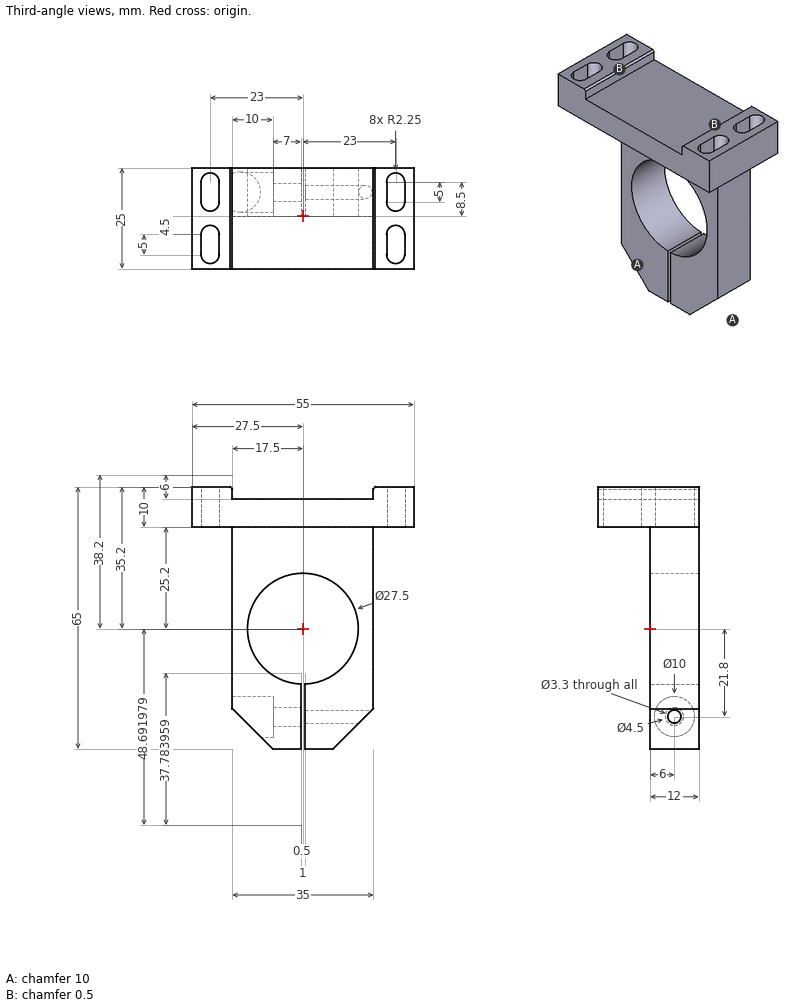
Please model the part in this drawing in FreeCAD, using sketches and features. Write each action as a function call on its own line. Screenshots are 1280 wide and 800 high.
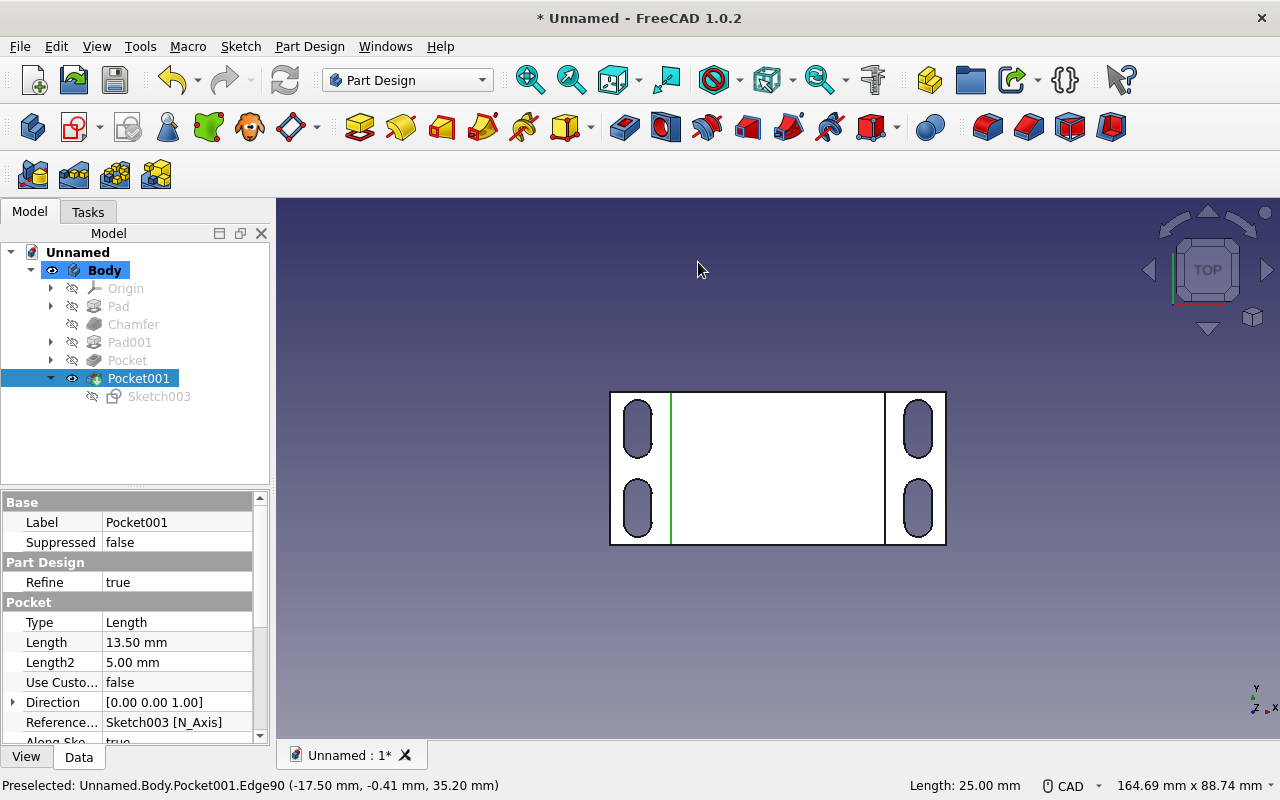
click(885, 467, ctrl)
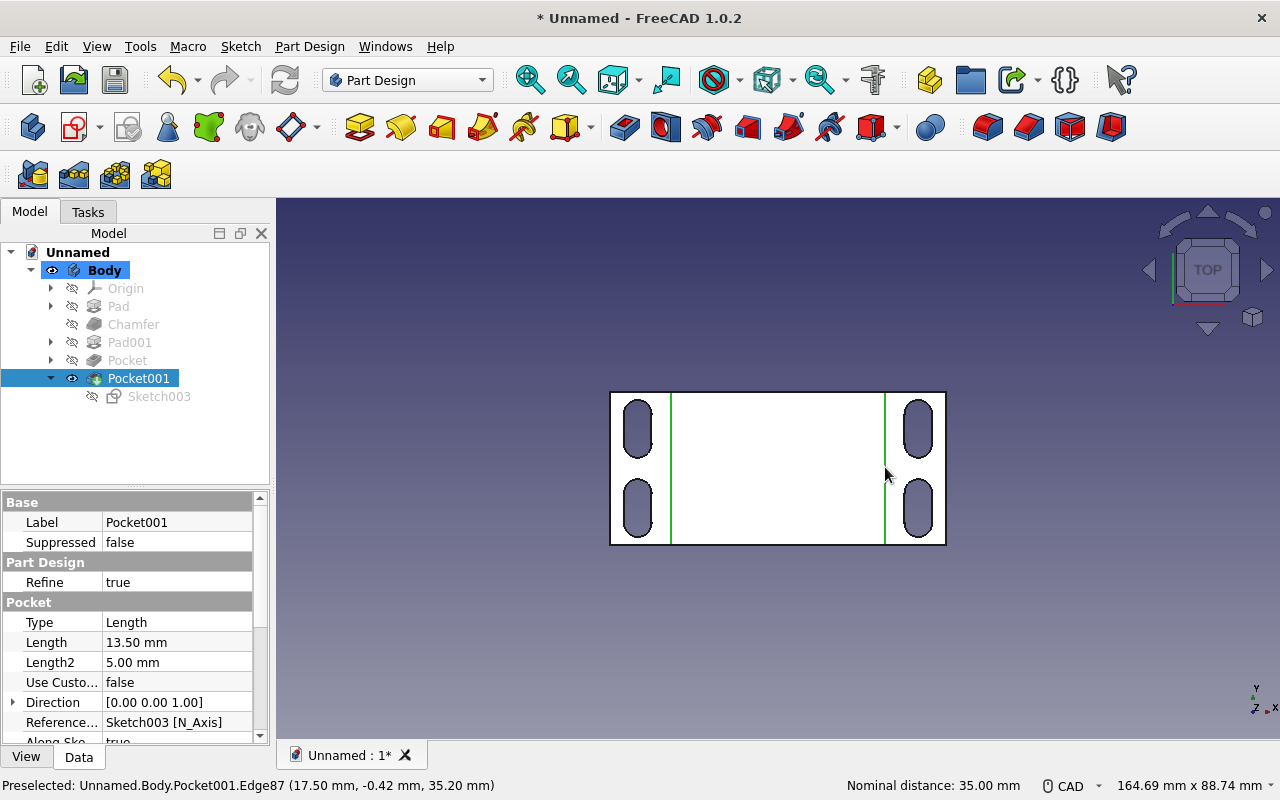
click(1029, 128)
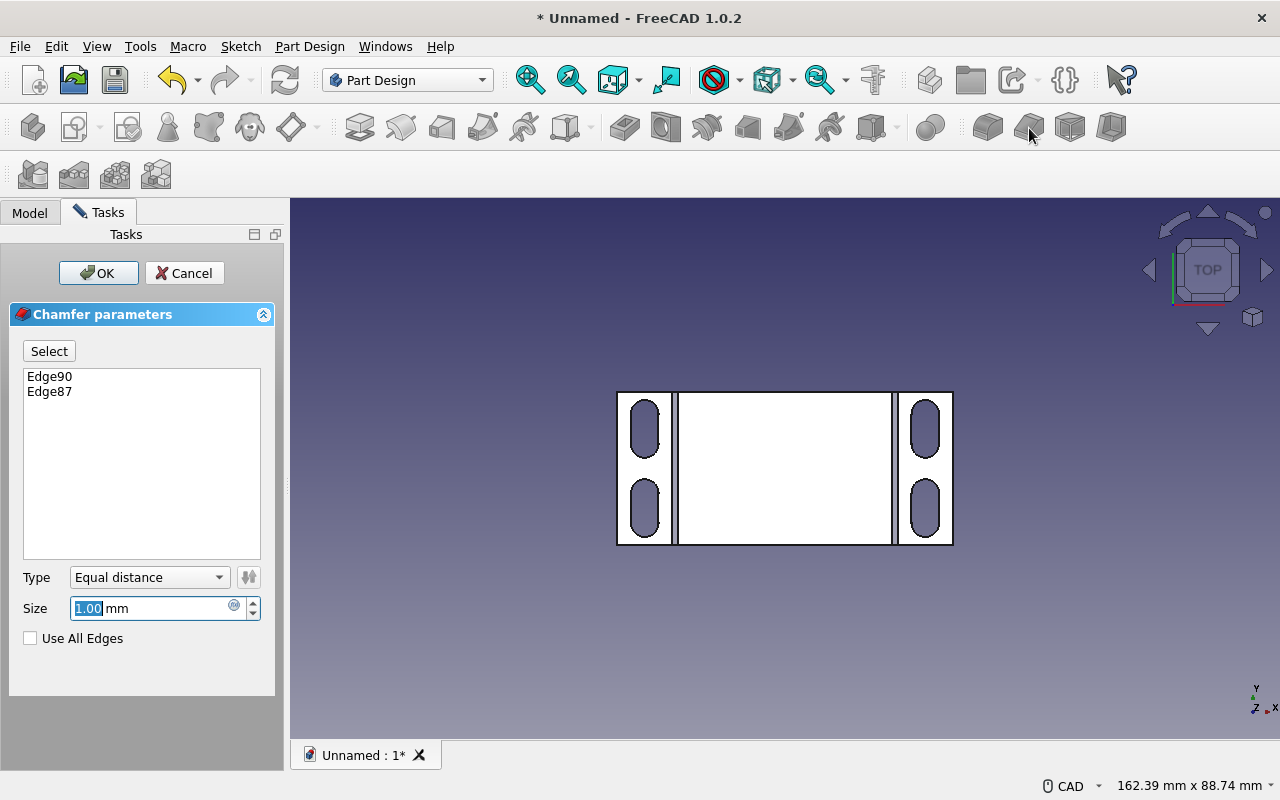
text(0.5)
key(Tab)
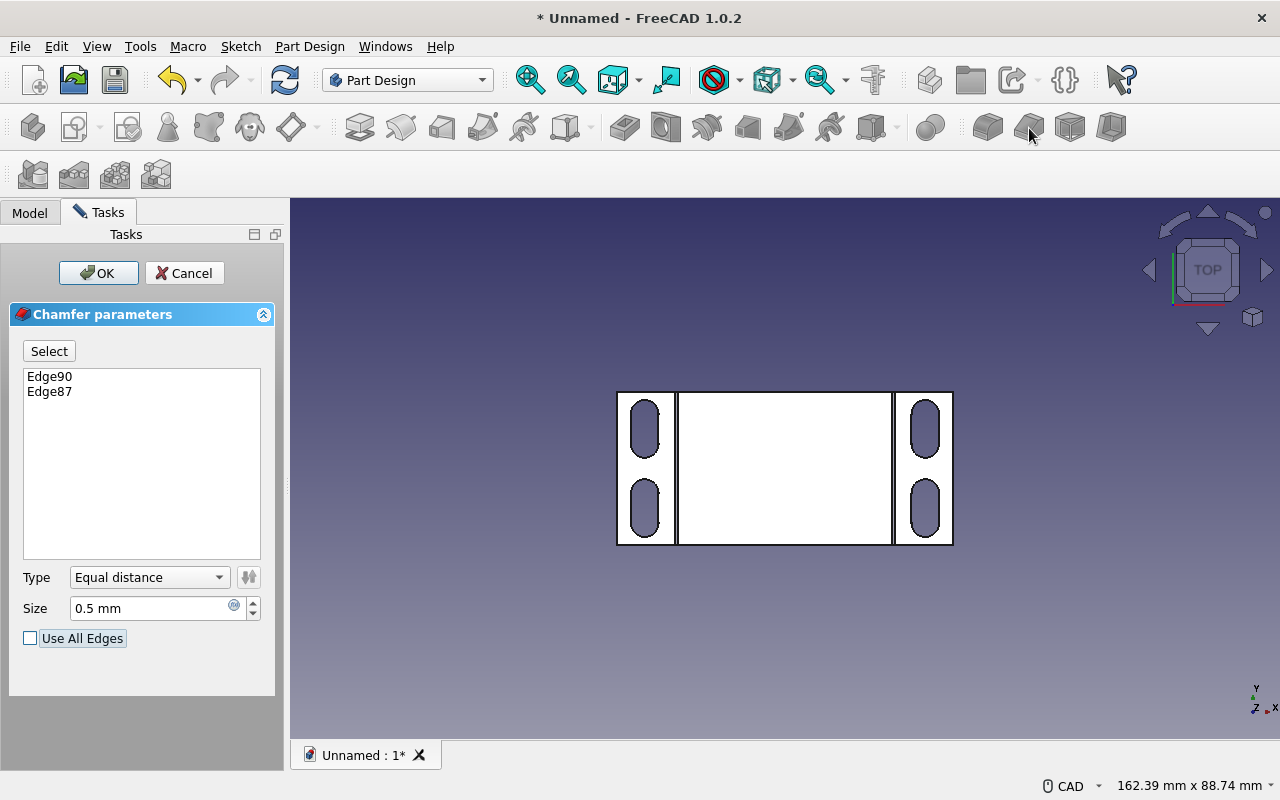
click(99, 273)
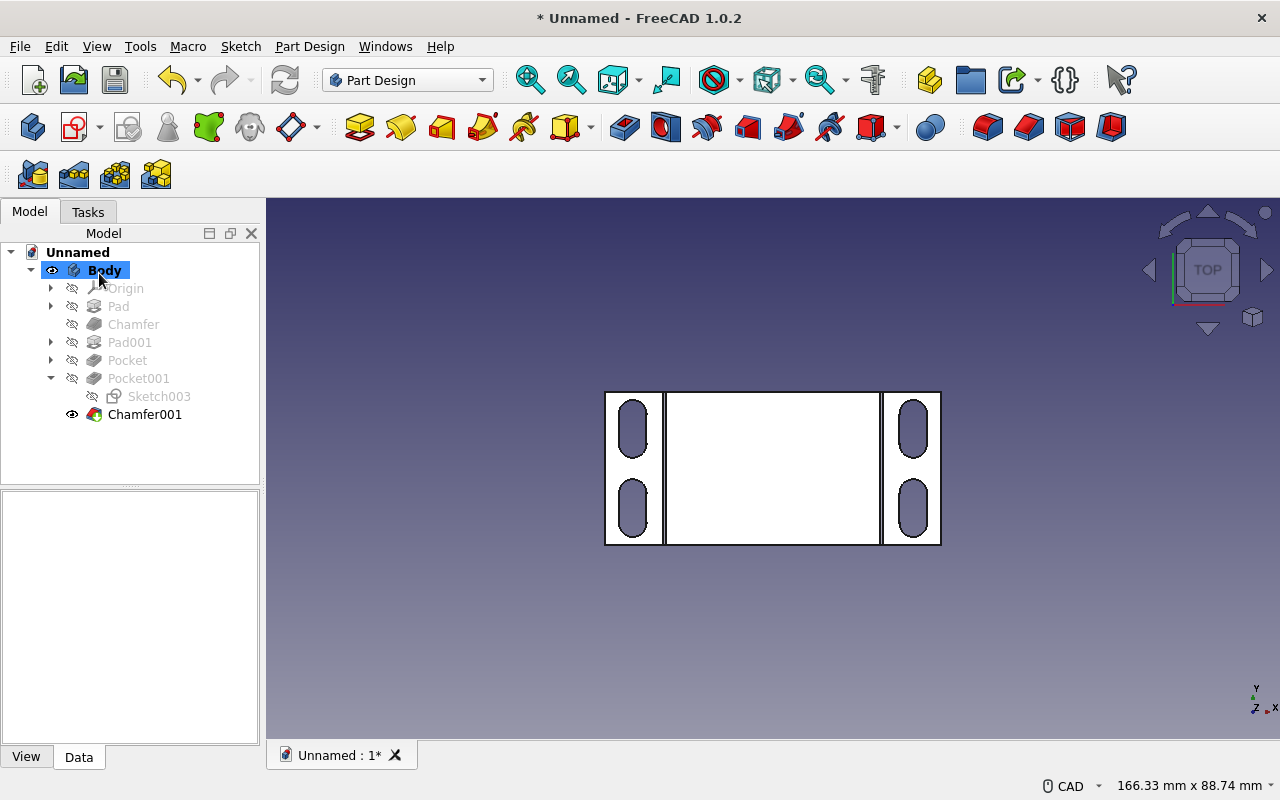
click(531, 80)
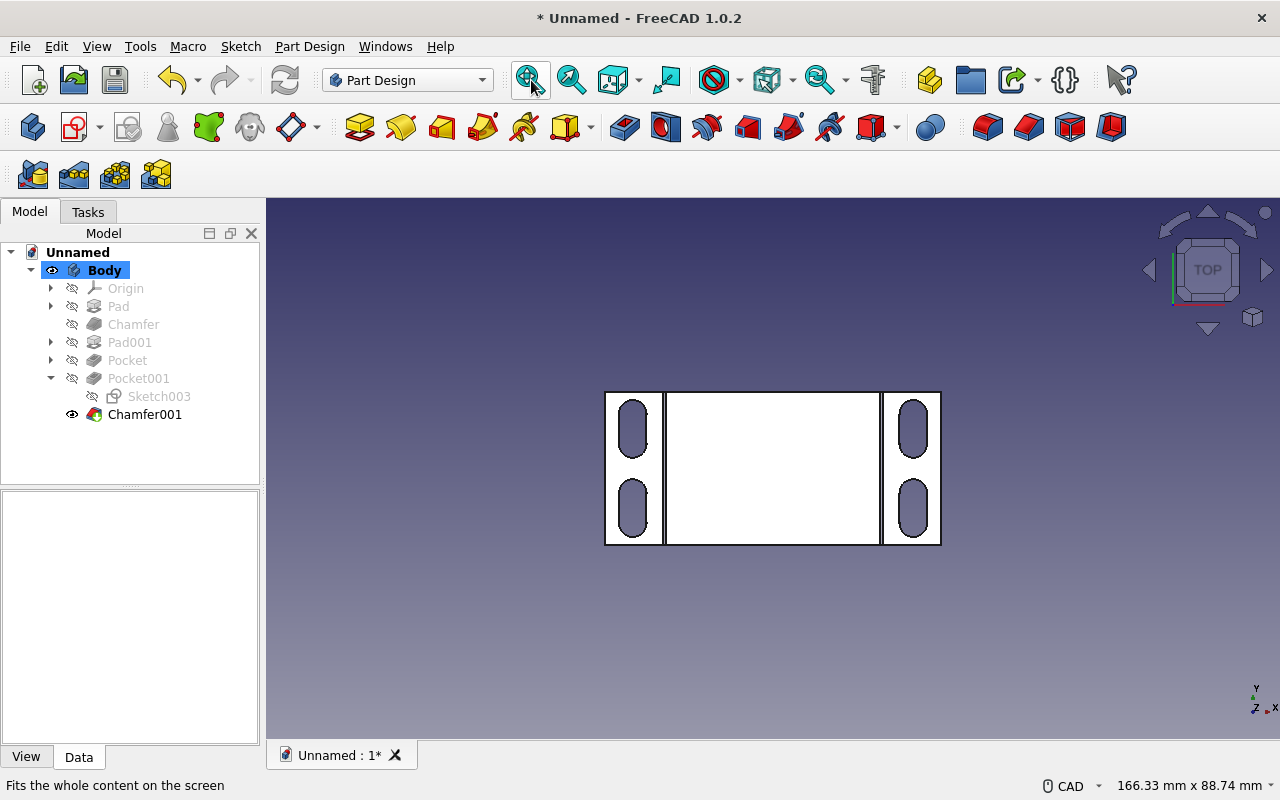
key(4)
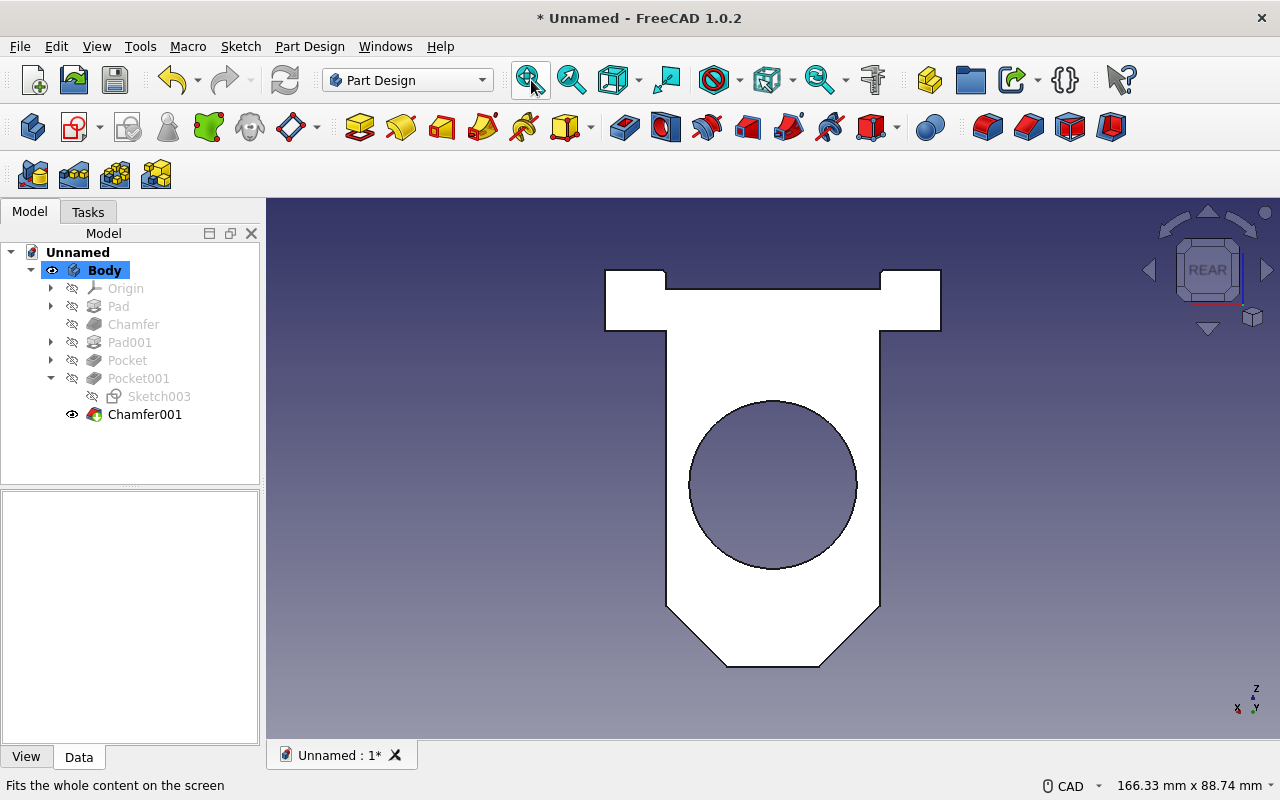
click(725, 354)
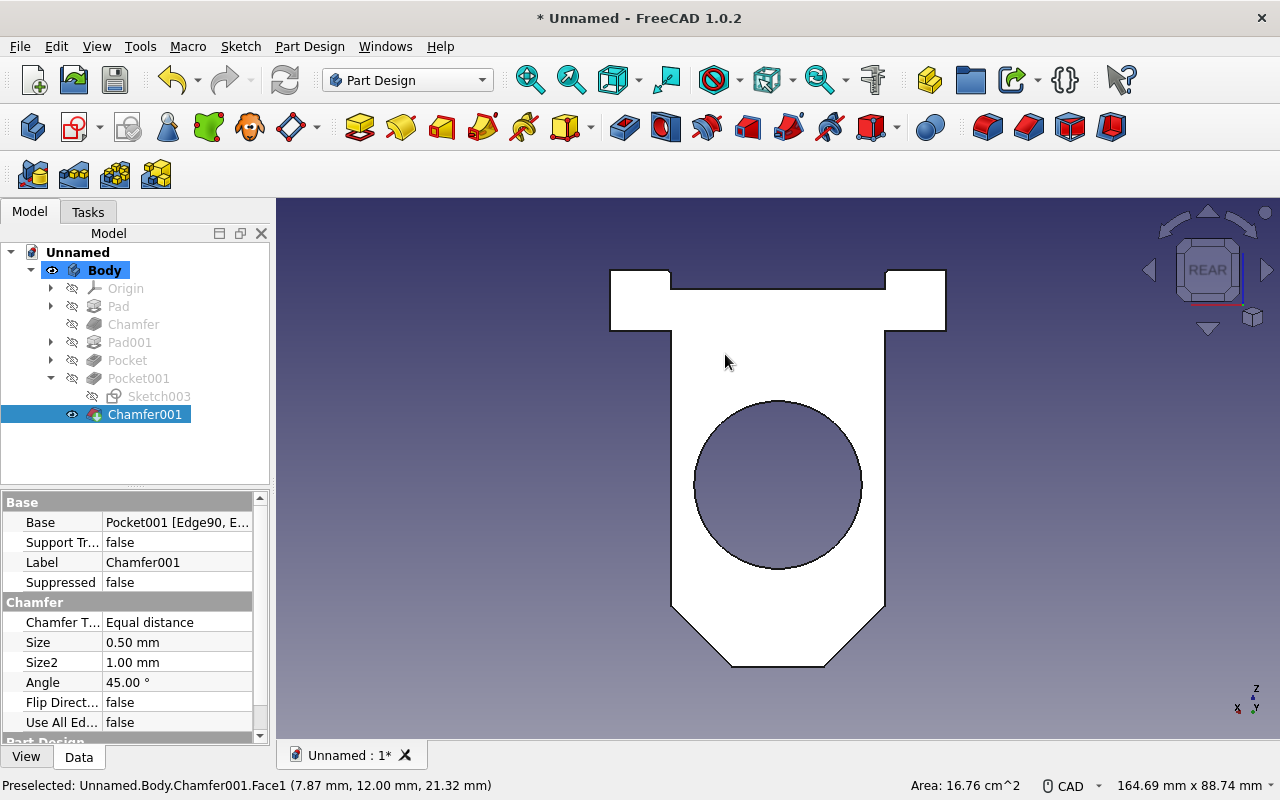
click(74, 128)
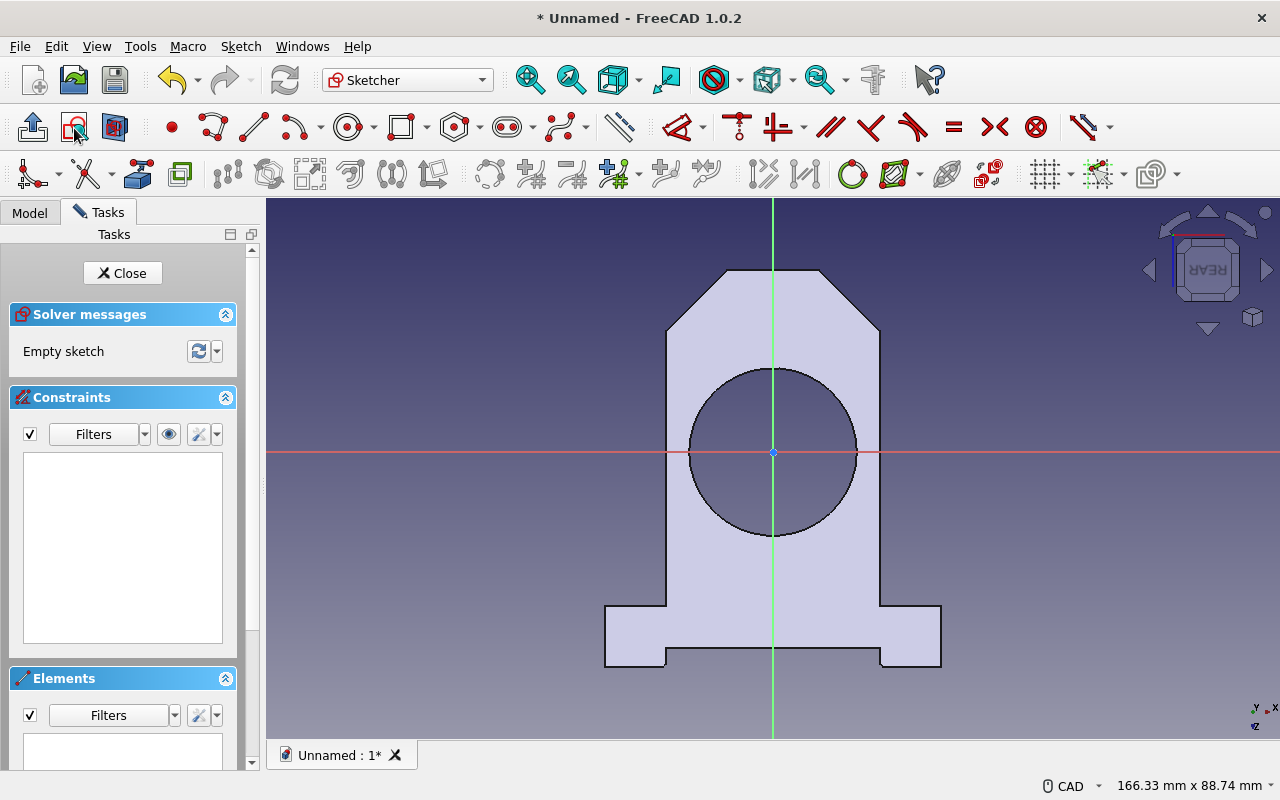
scroll(395, 711, down, 1)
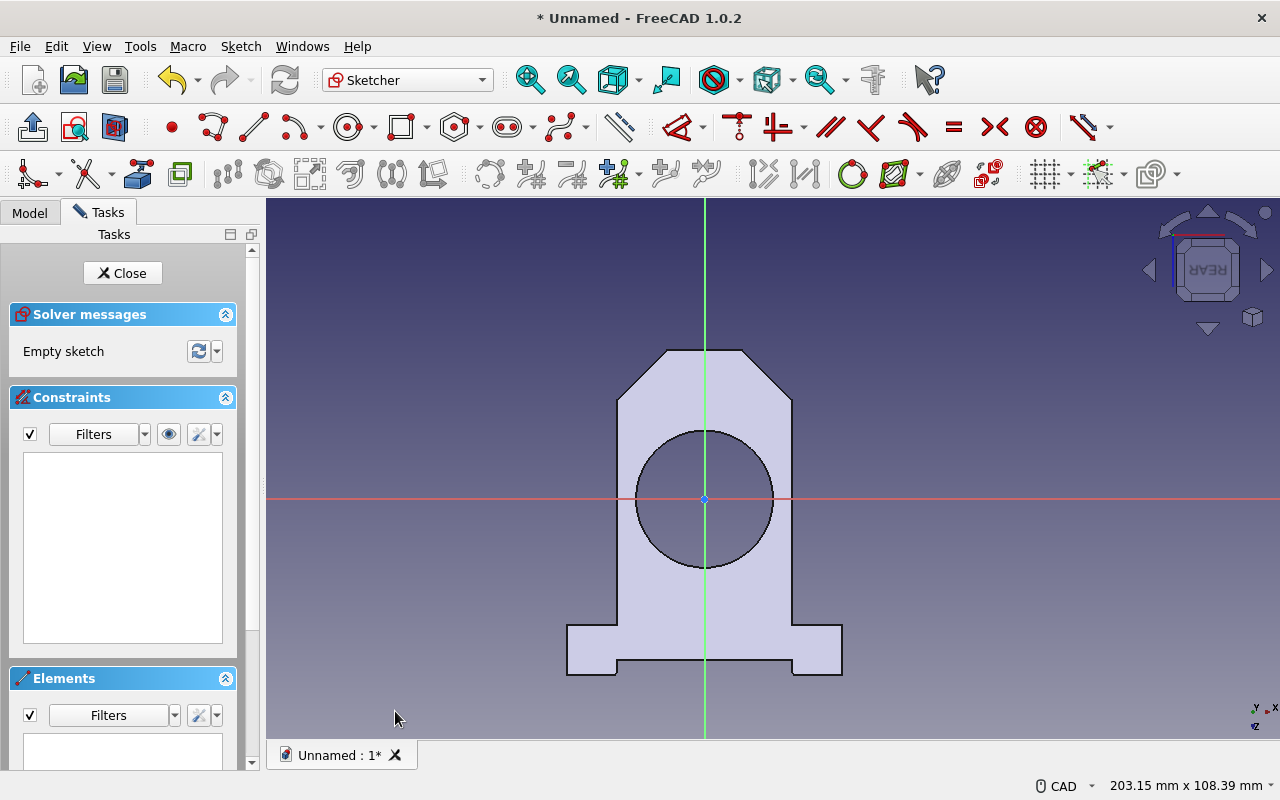
scroll(705, 226, up, 2)